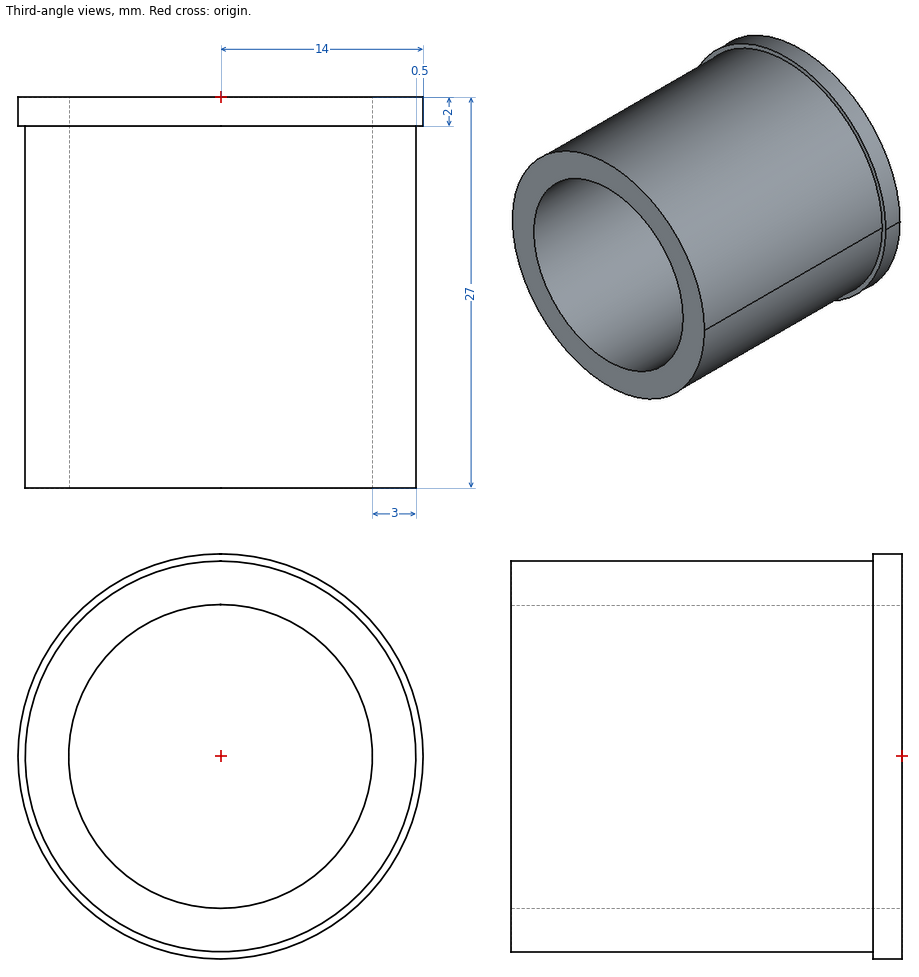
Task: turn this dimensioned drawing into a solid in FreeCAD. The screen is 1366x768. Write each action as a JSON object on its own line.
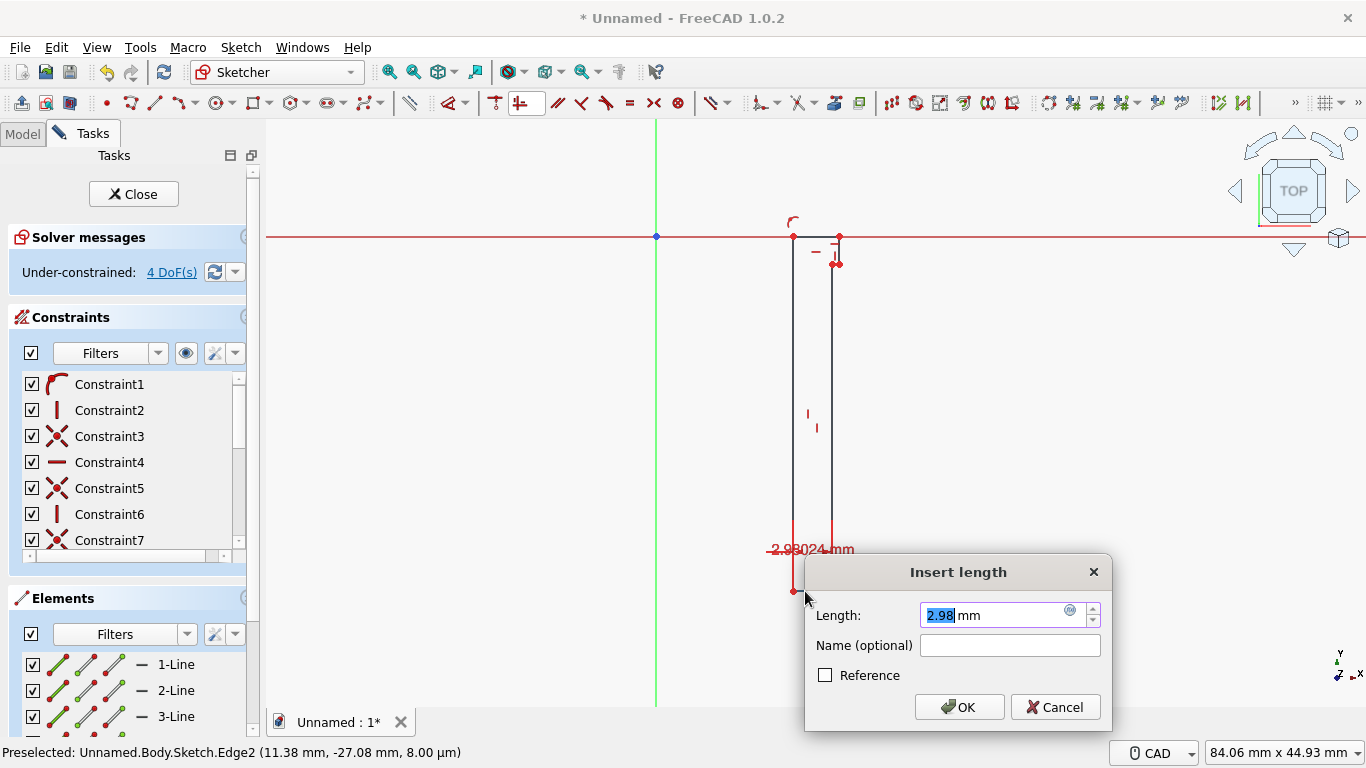
{"action": "type", "text": "3"}
{"action": "key", "text": "Return"}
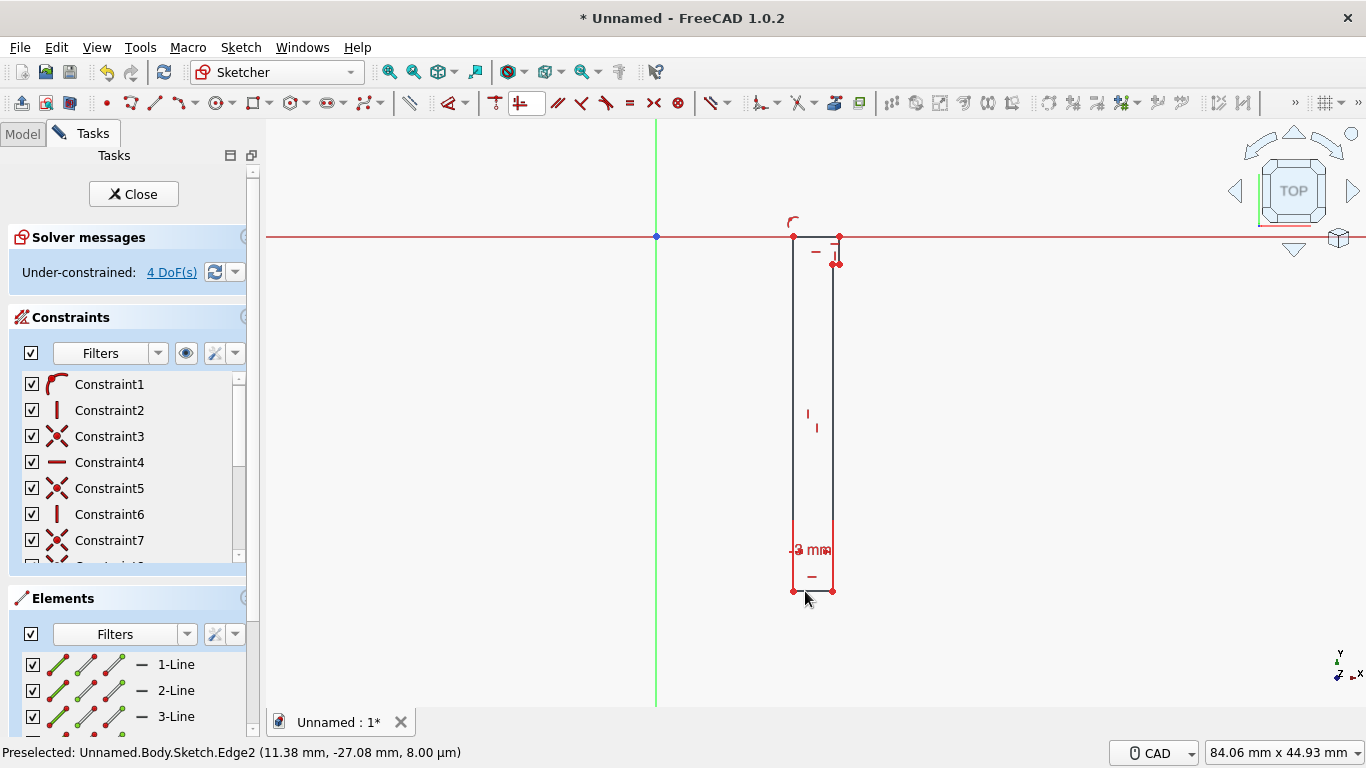
{"action": "scroll", "coordinate": [839, 253], "scroll_direction": "up", "scroll_amount": 3}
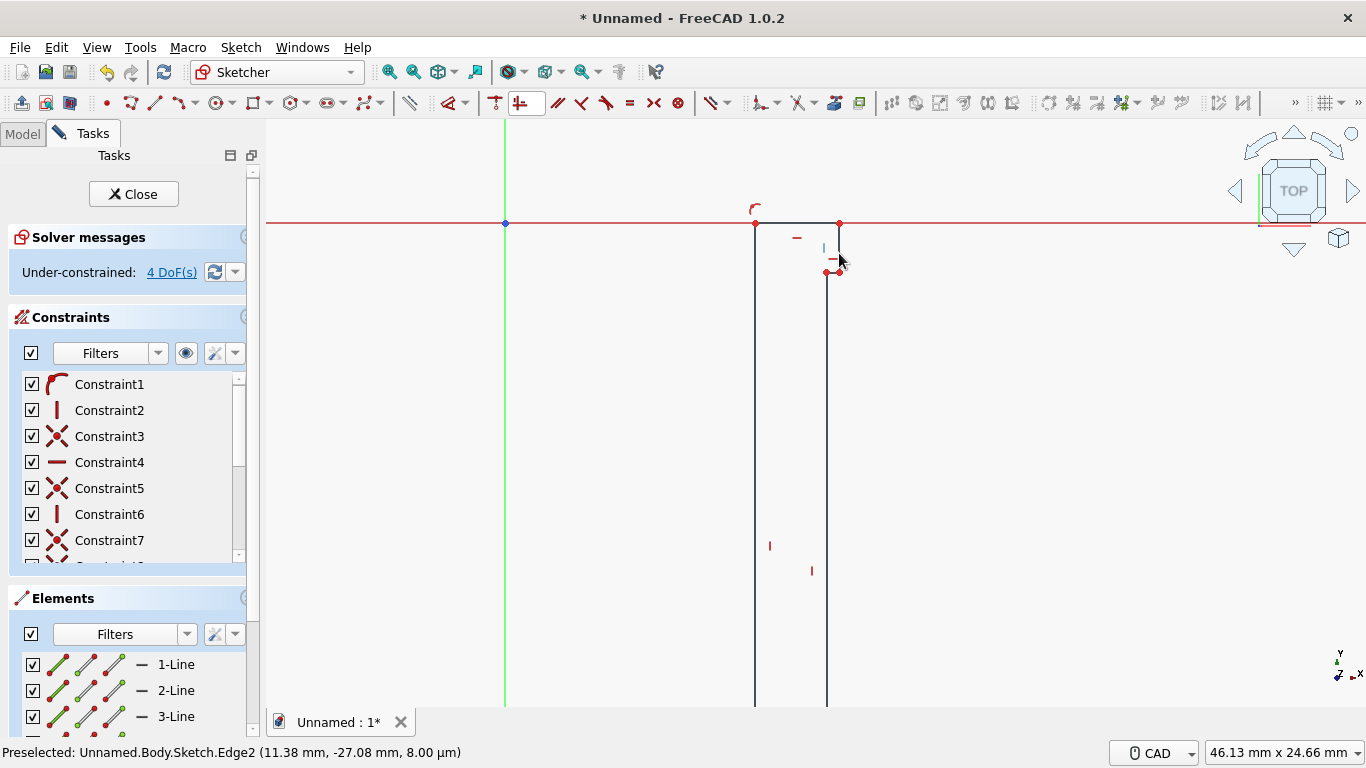
{"action": "left_click", "coordinate": [839, 243]}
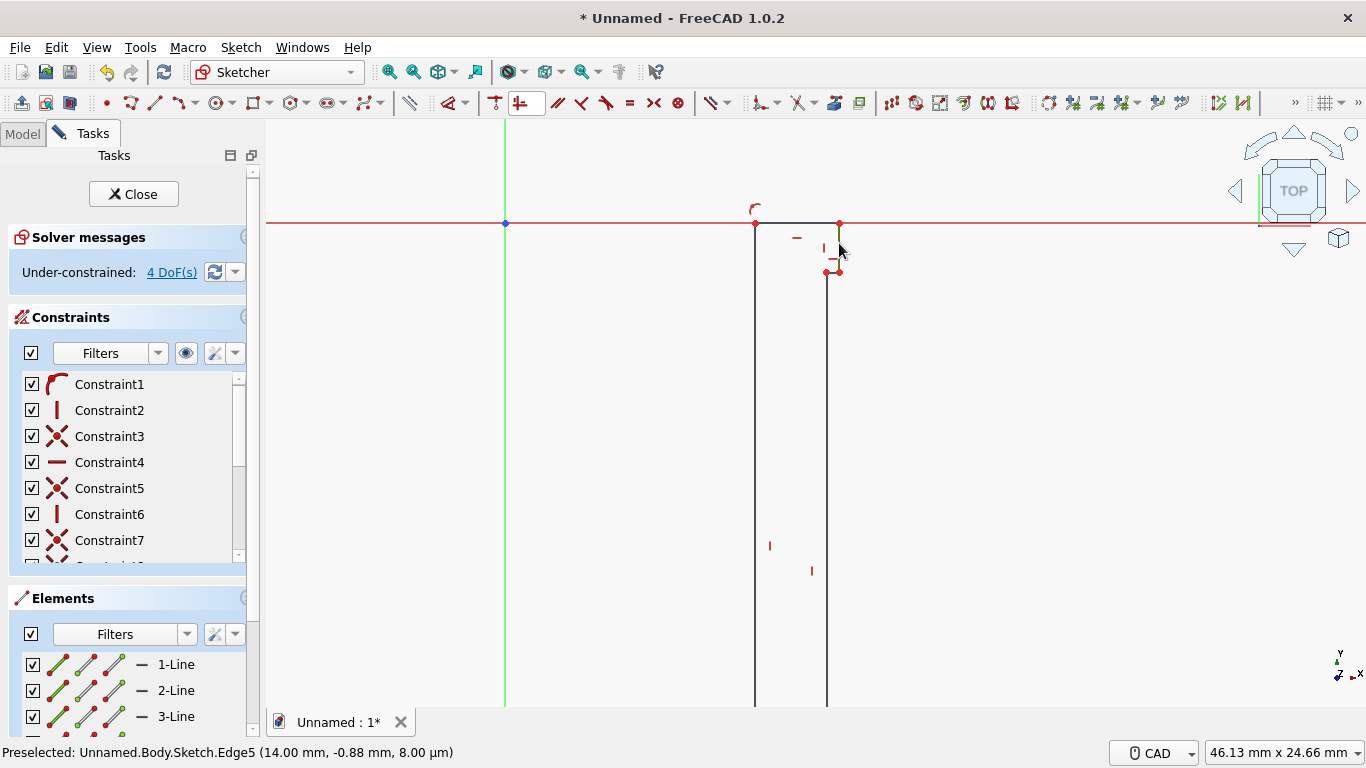
{"action": "key", "text": "i"}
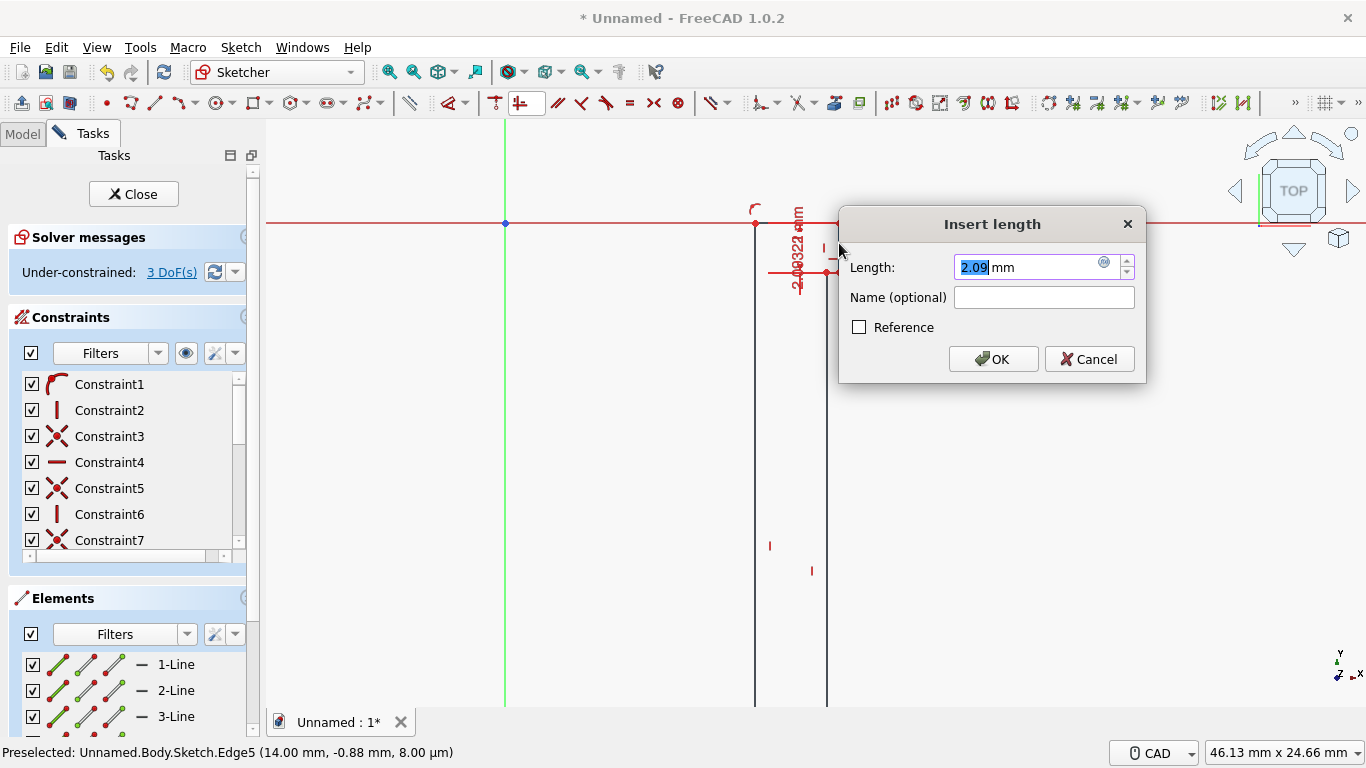
{"action": "type", "text": "2"}
{"action": "key", "text": "Return"}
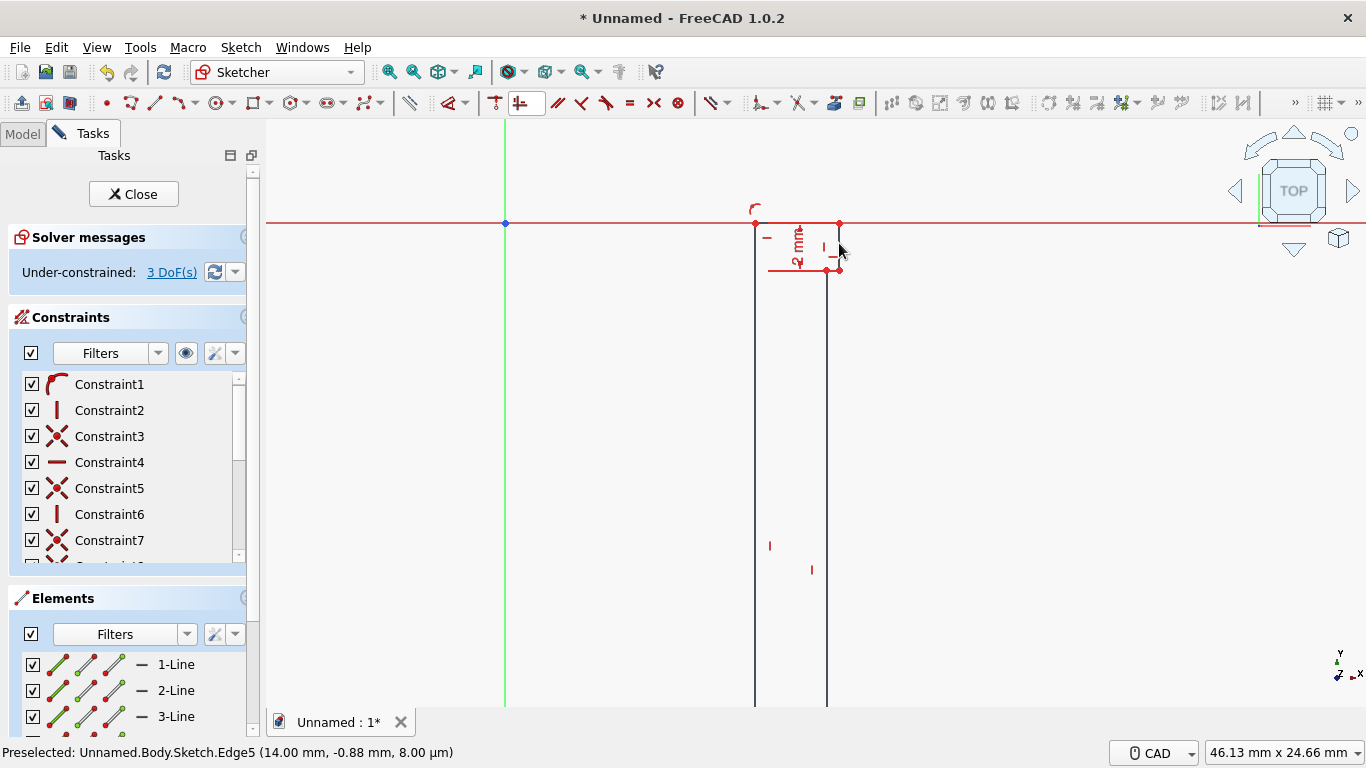
{"action": "left_click", "coordinate": [755, 417]}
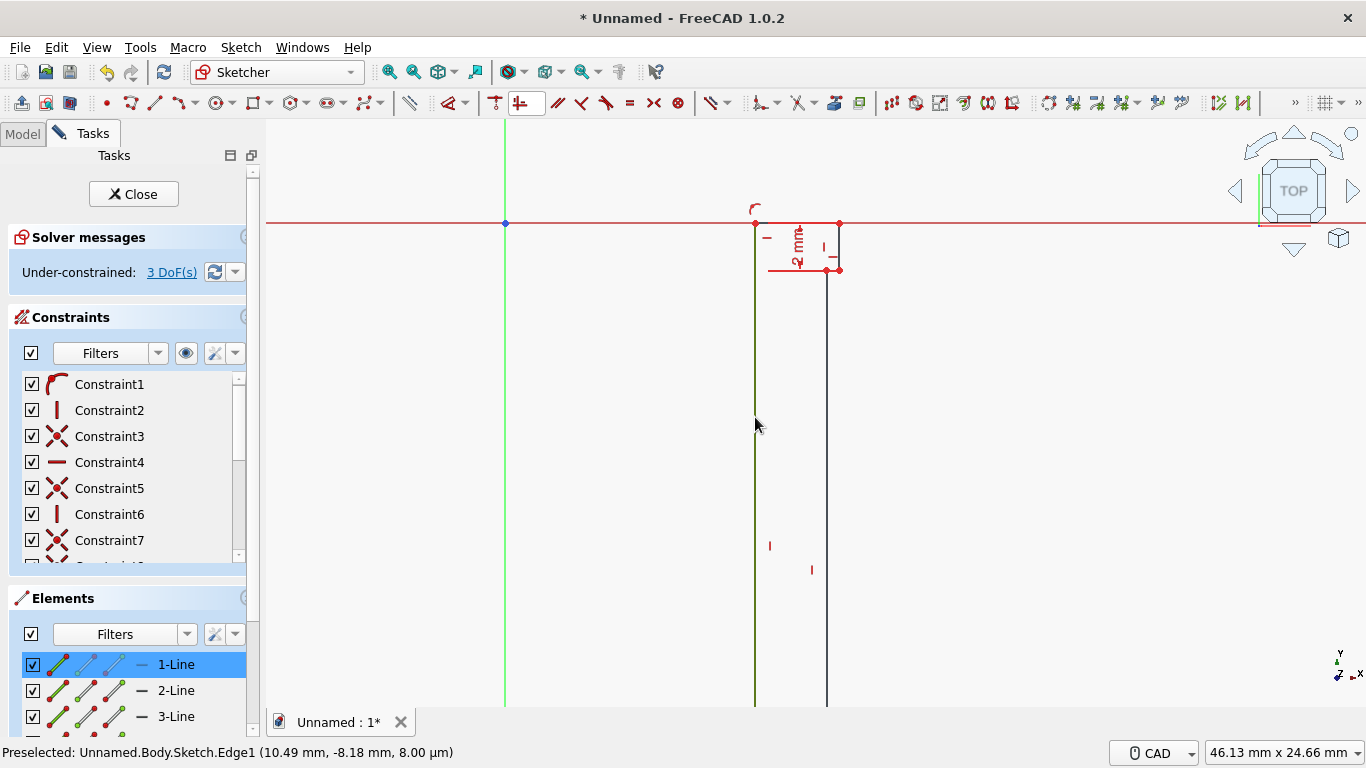
{"action": "left_click", "coordinate": [468, 104]}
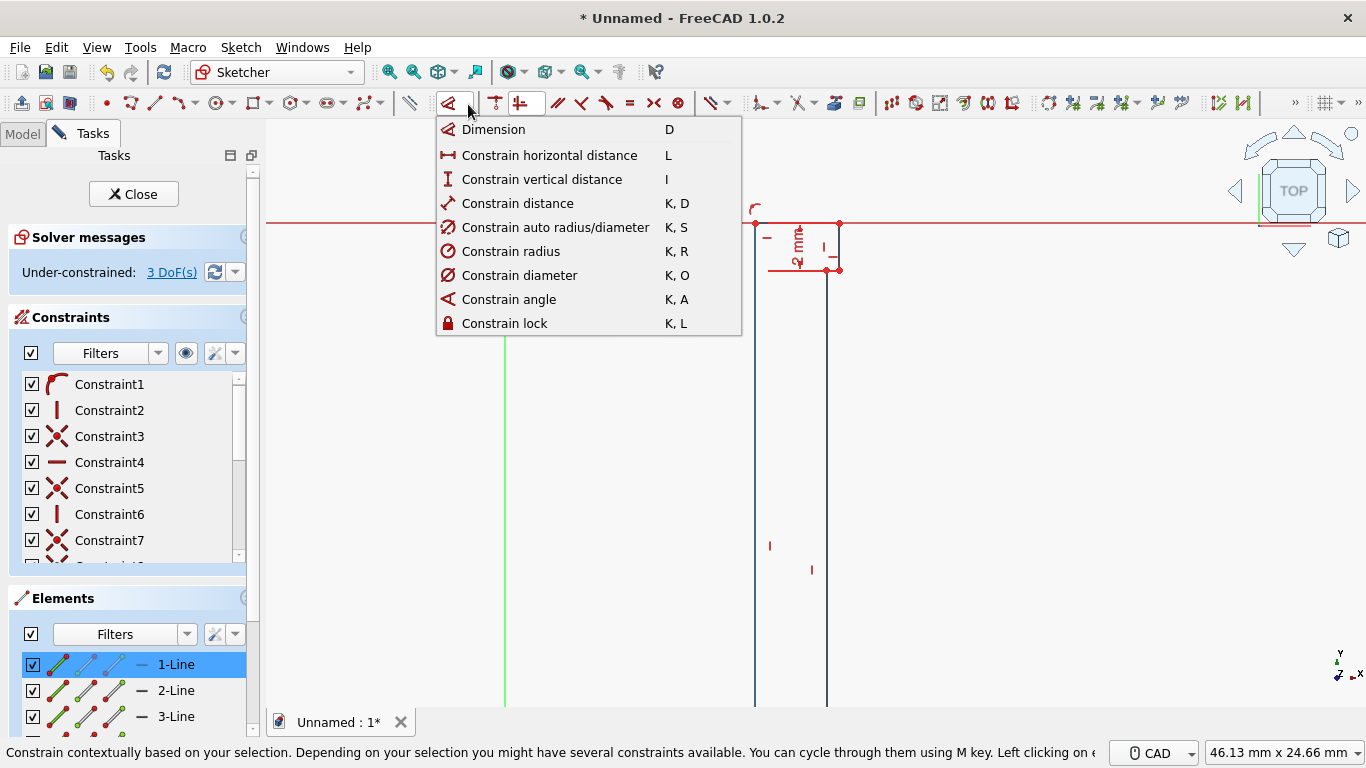
{"action": "left_click", "coordinate": [589, 179]}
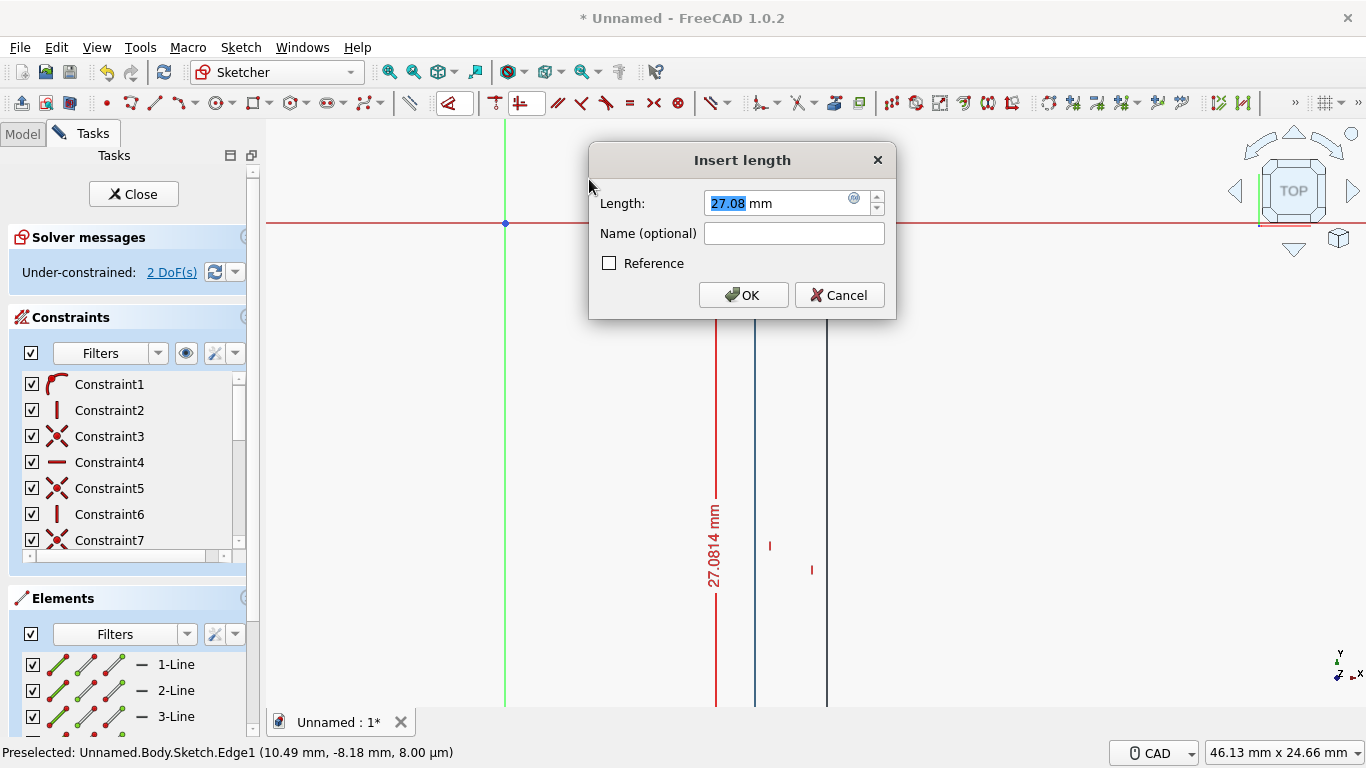
{"action": "type", "text": "27"}
{"action": "key", "text": "Return"}